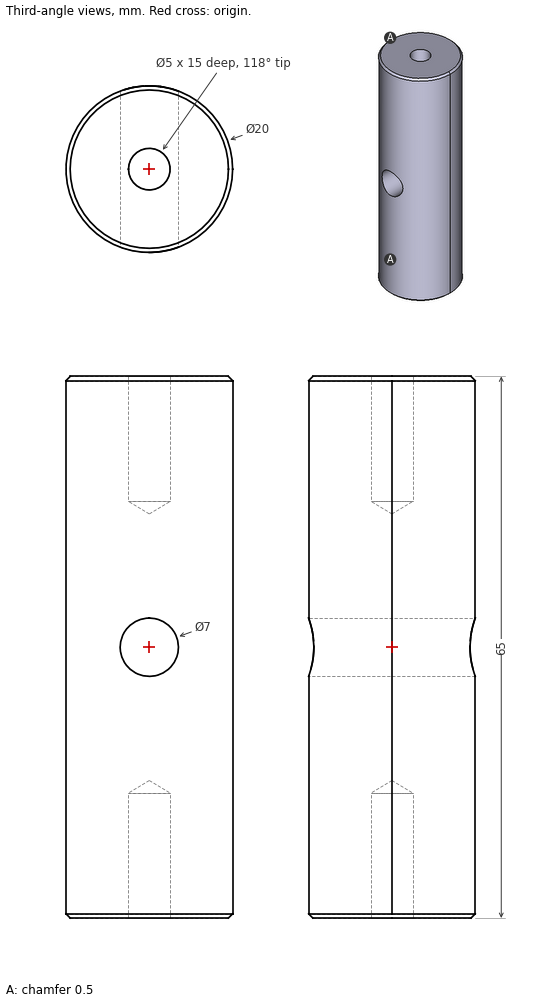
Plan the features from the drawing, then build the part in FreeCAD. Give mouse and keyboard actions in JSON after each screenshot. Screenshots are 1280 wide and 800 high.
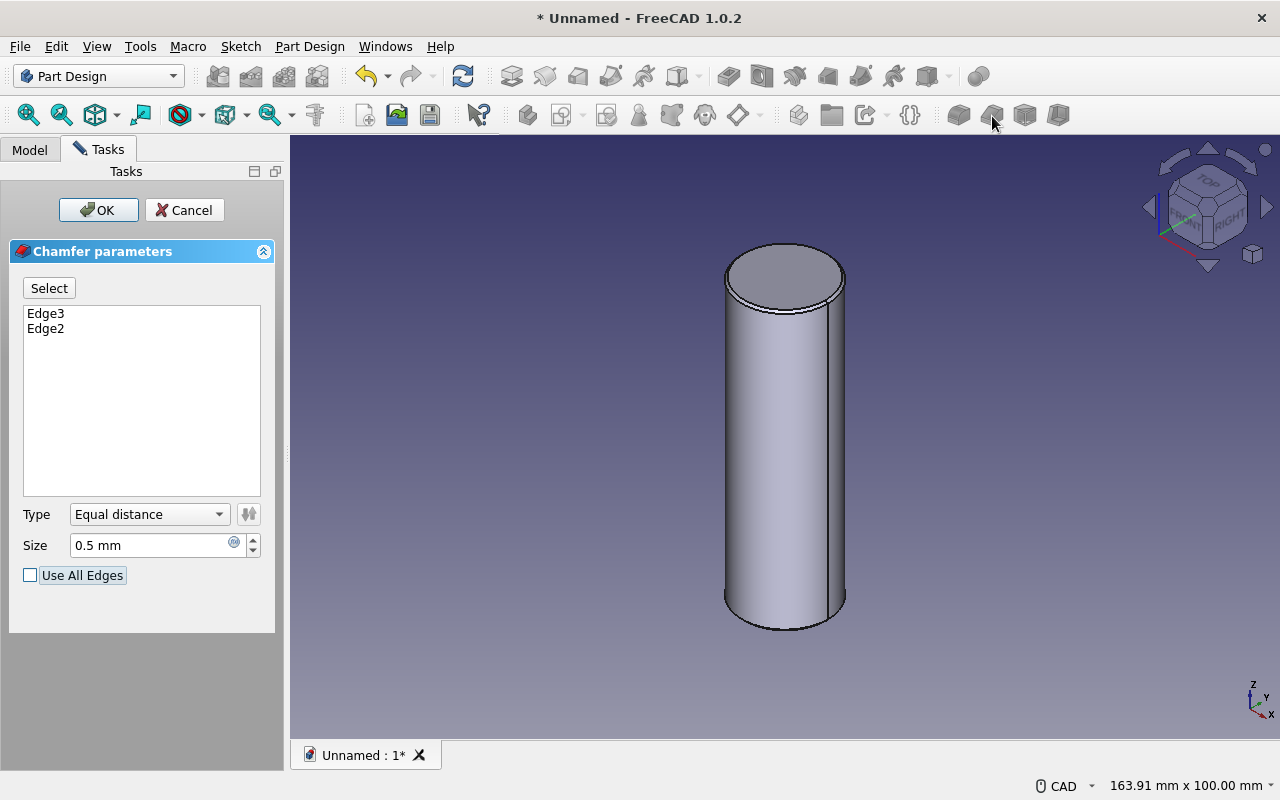
{"action": "left_click", "coordinate": [99, 210]}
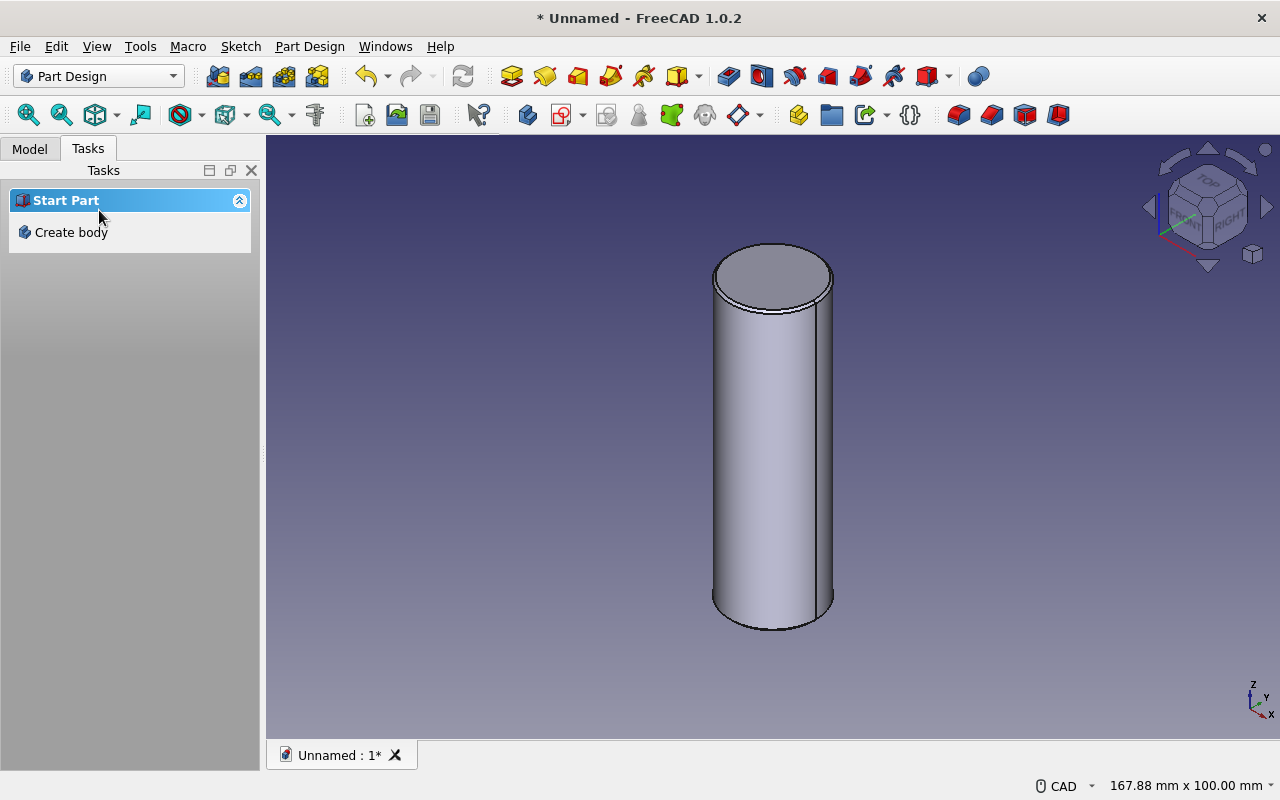
{"action": "left_click", "coordinate": [773, 276]}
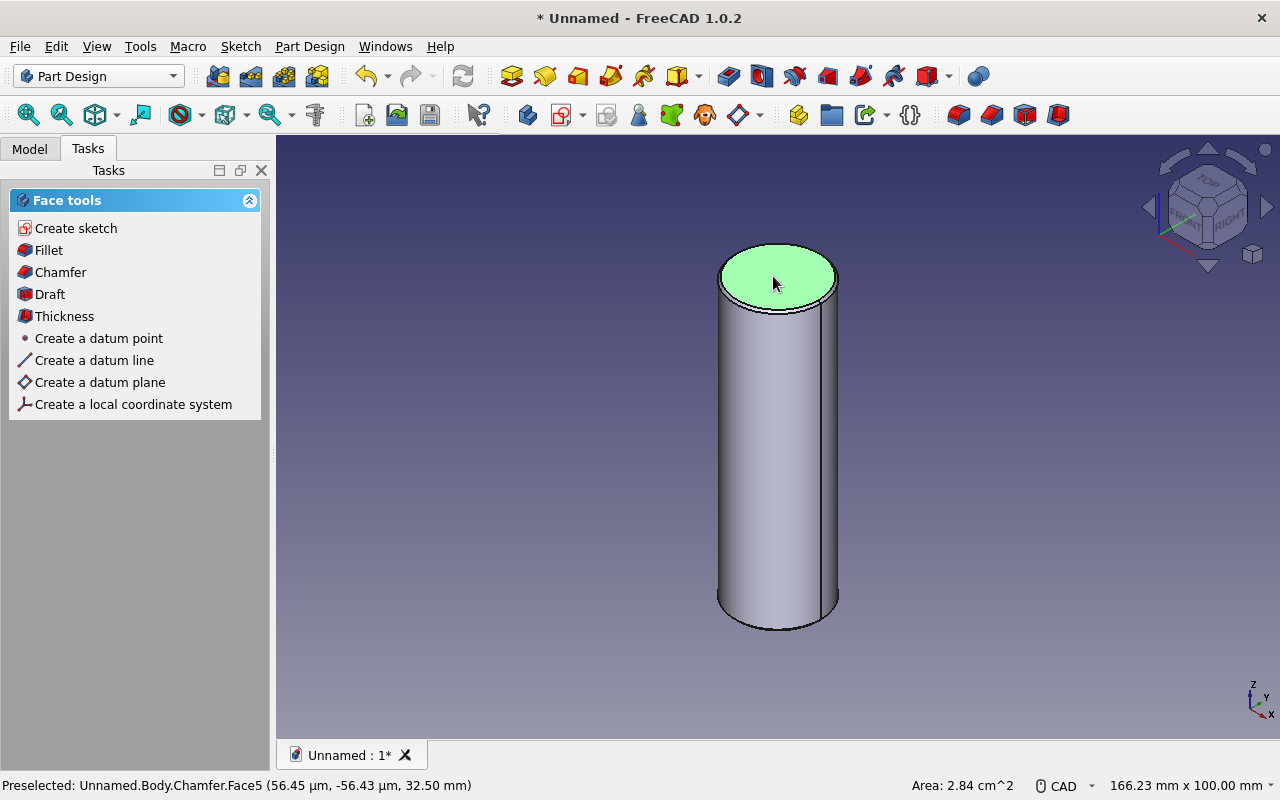
{"action": "left_click", "coordinate": [560, 116]}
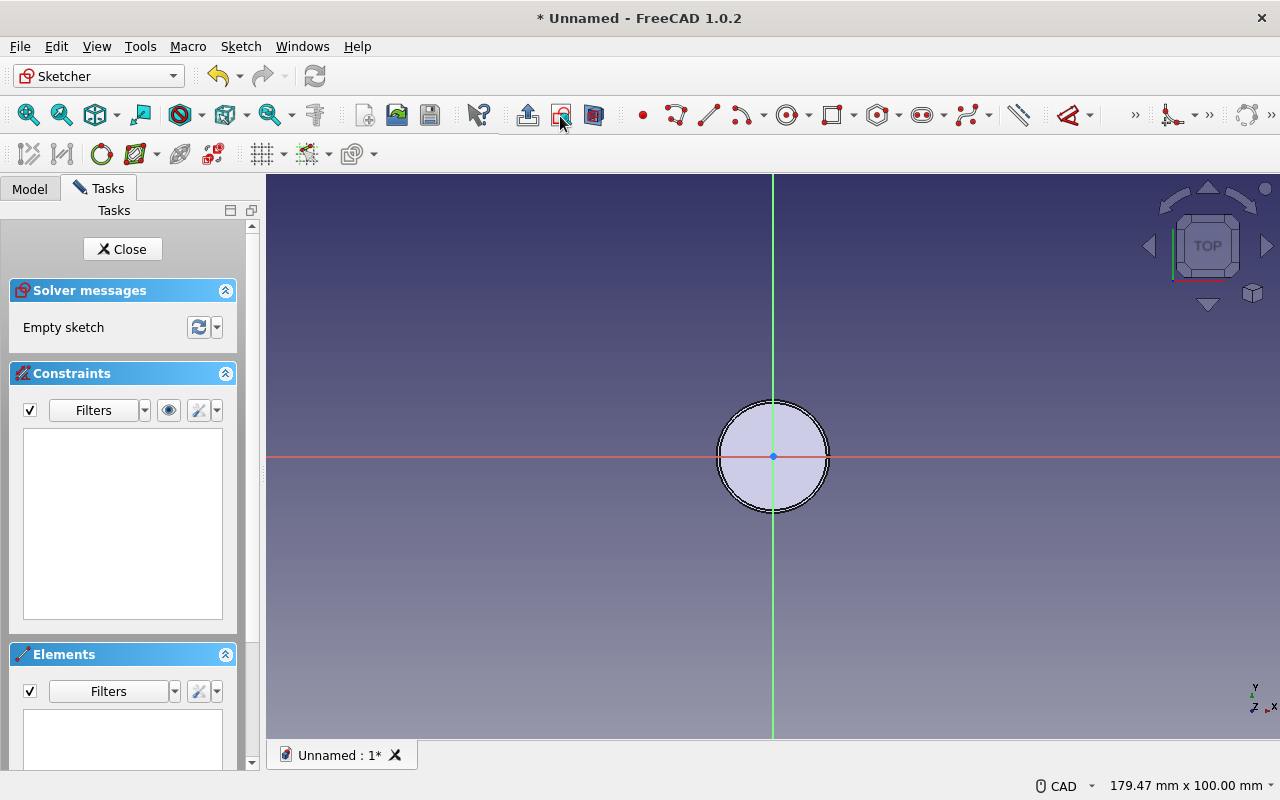
{"action": "scroll", "coordinate": [778, 456], "scroll_direction": "up", "scroll_amount": 13}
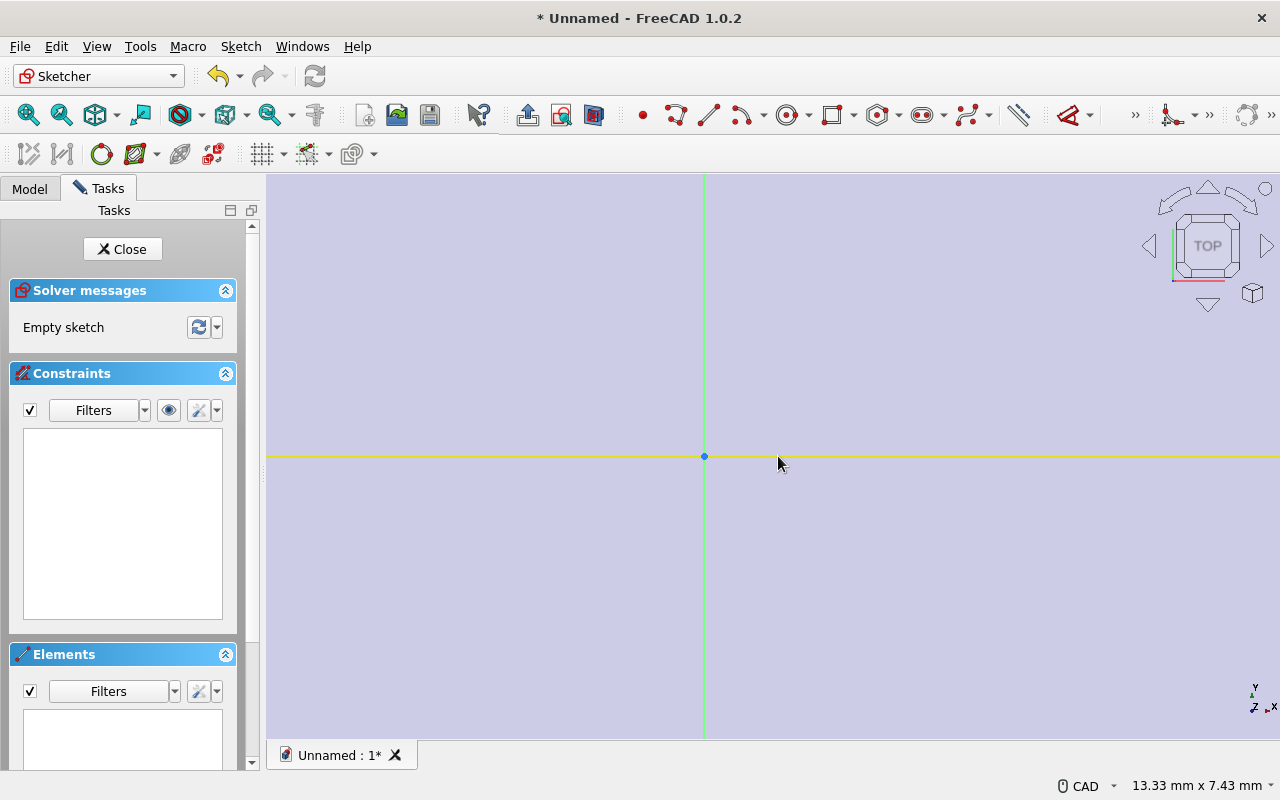
{"action": "left_click", "coordinate": [786, 116]}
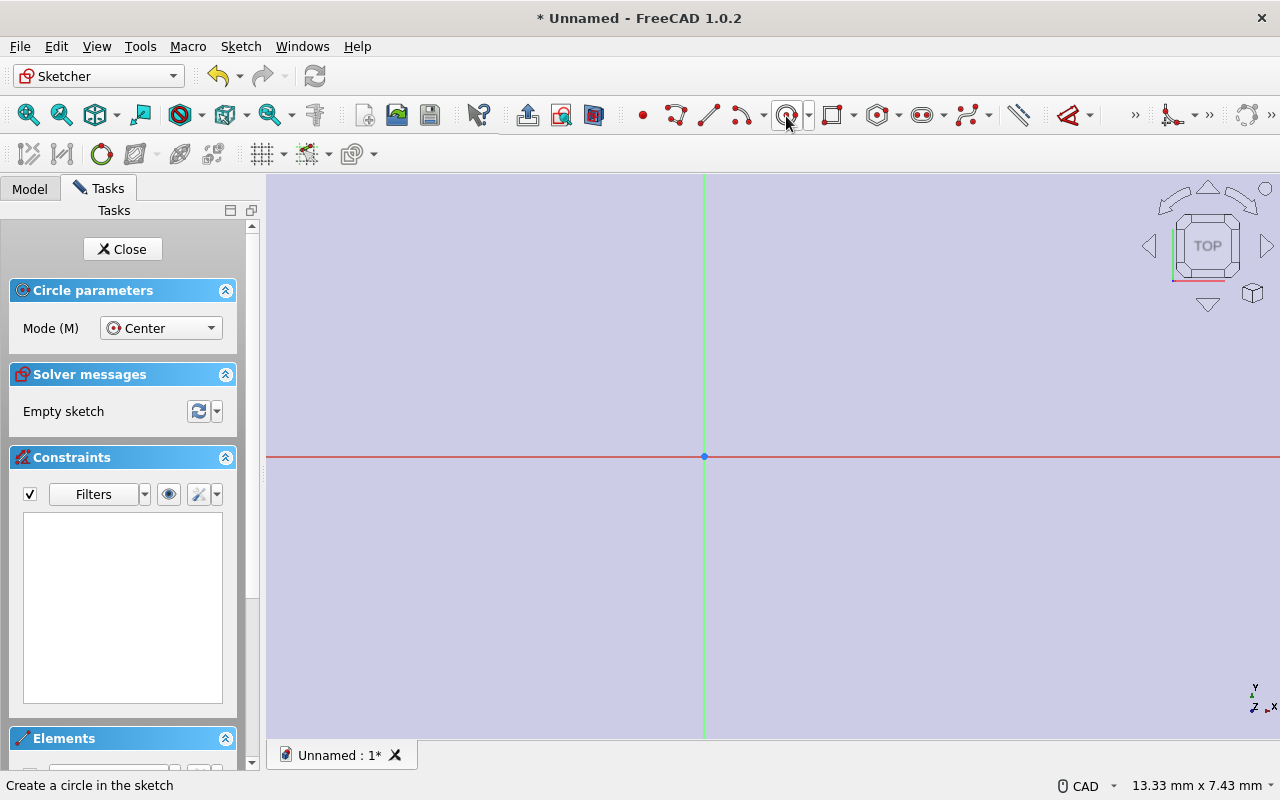
{"action": "left_click", "coordinate": [704, 456]}
{"action": "left_click", "coordinate": [839, 322]}
{"action": "key", "text": "Escape"}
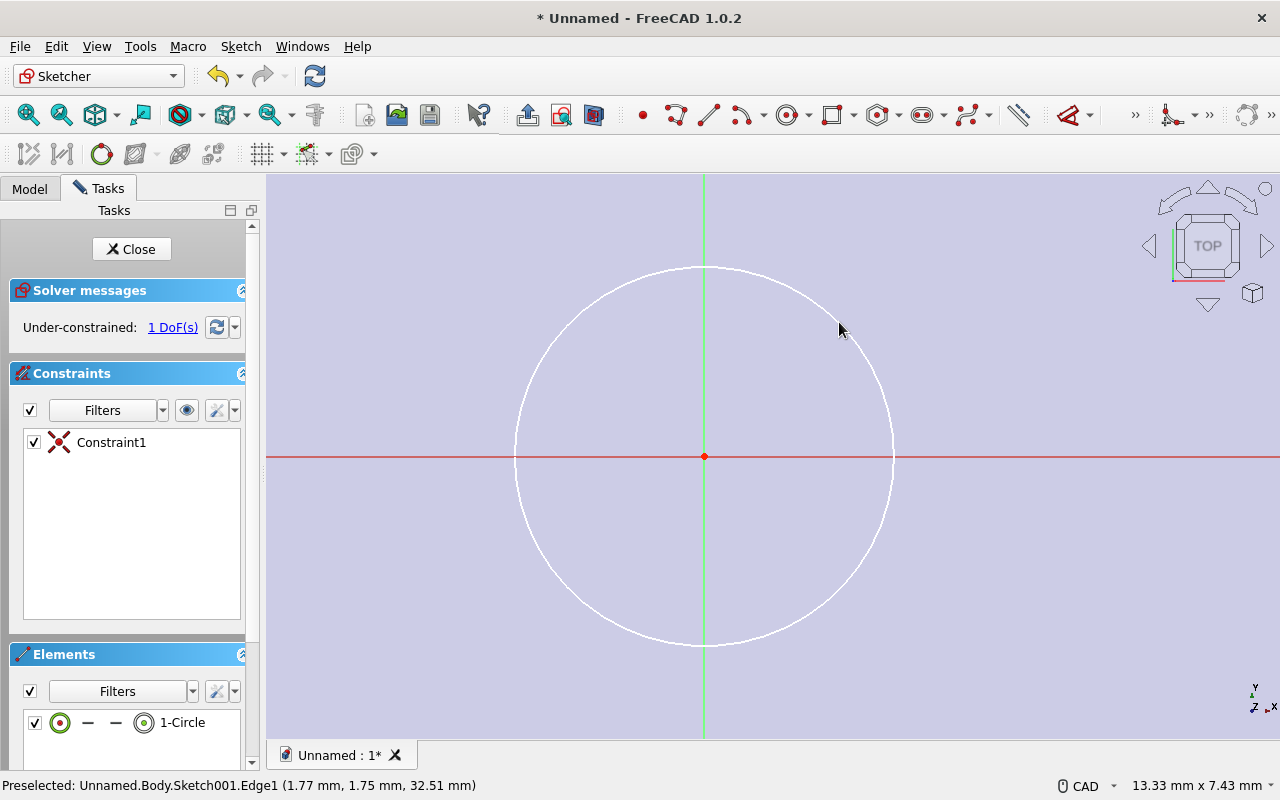
{"action": "left_click", "coordinate": [1068, 116]}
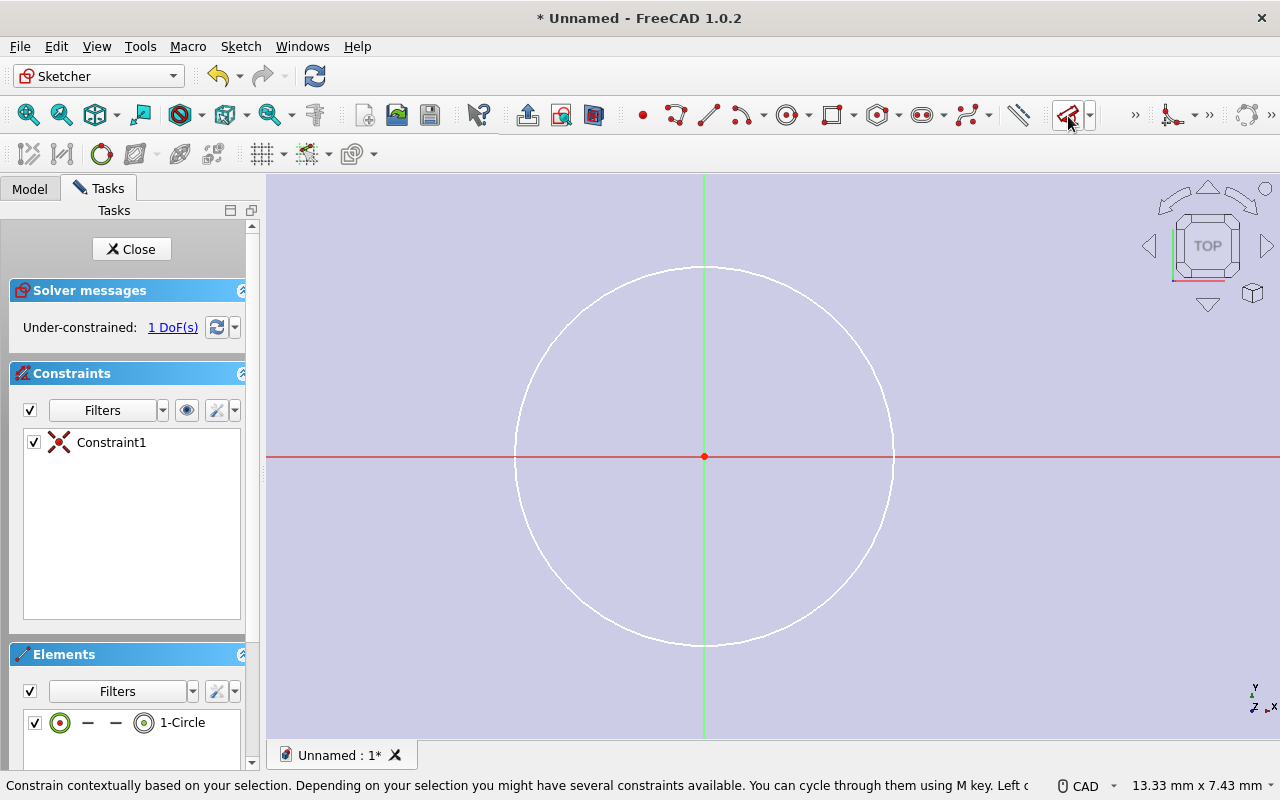
{"action": "left_click", "coordinate": [838, 322]}
{"action": "left_click", "coordinate": [861, 299]}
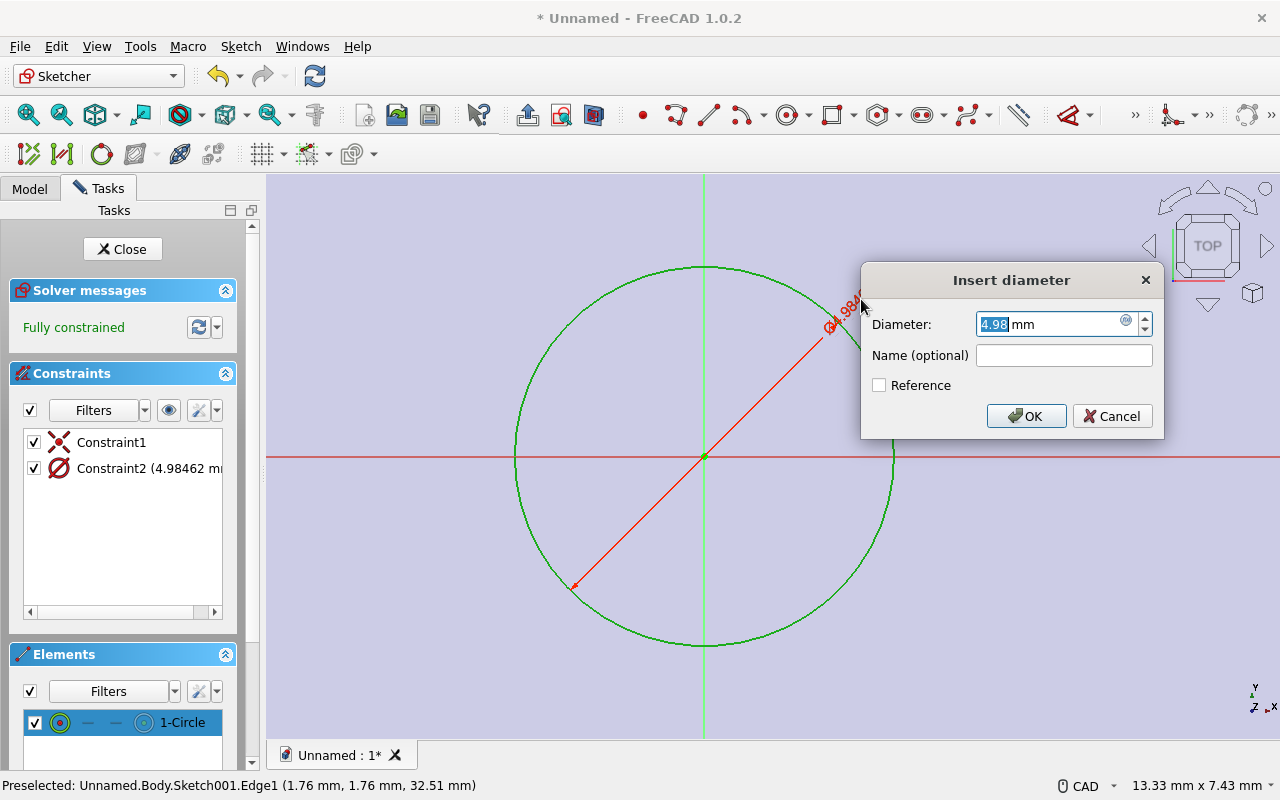
{"action": "type", "text": "5"}
{"action": "key", "text": "Return"}
{"action": "key", "text": "Escape"}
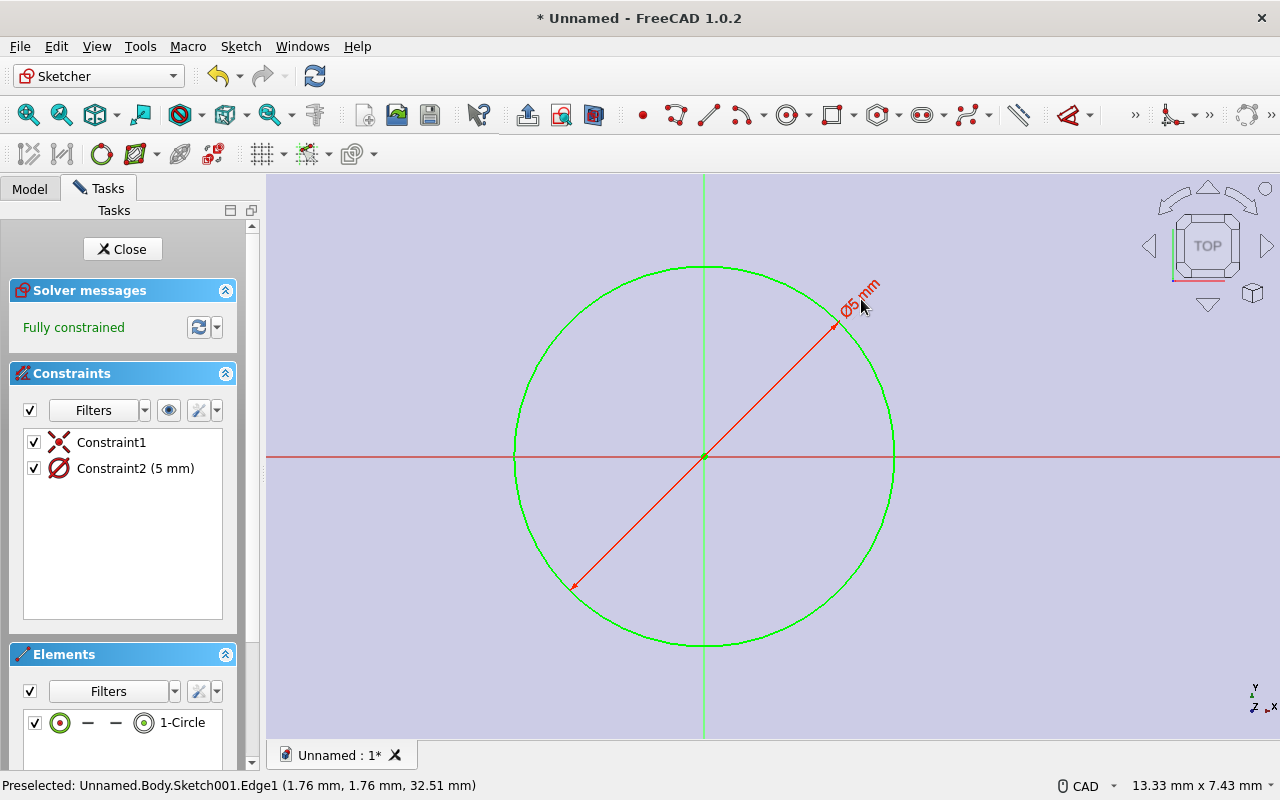
{"action": "left_click", "coordinate": [123, 249]}